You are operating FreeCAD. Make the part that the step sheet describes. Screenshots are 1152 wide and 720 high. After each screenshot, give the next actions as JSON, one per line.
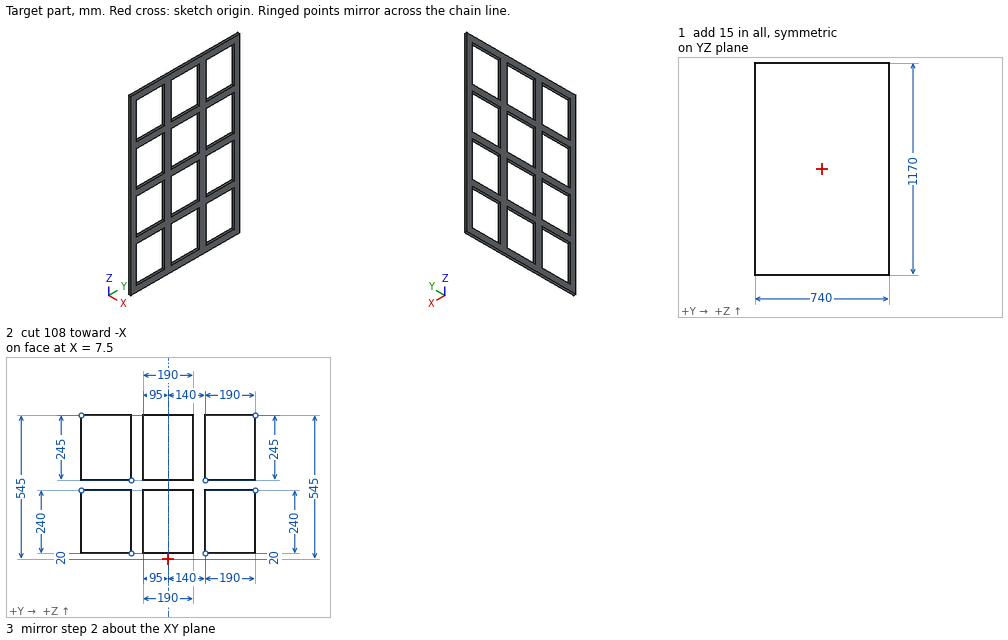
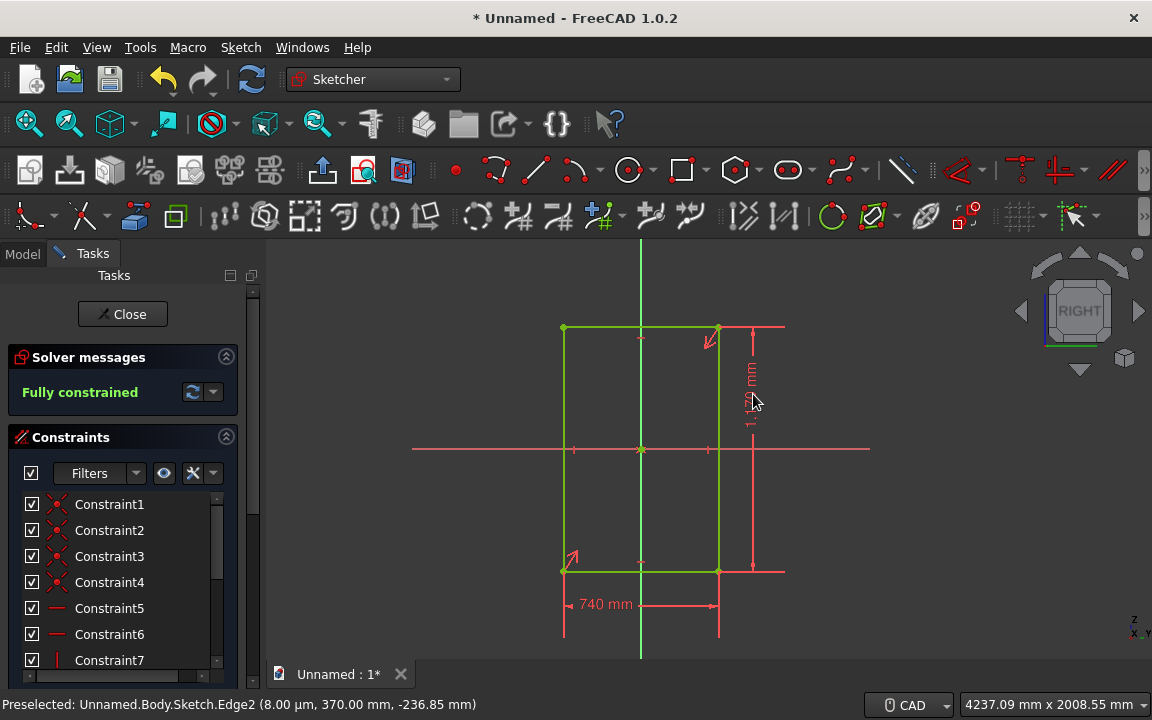
{"action": "left_click", "coordinate": [123, 314]}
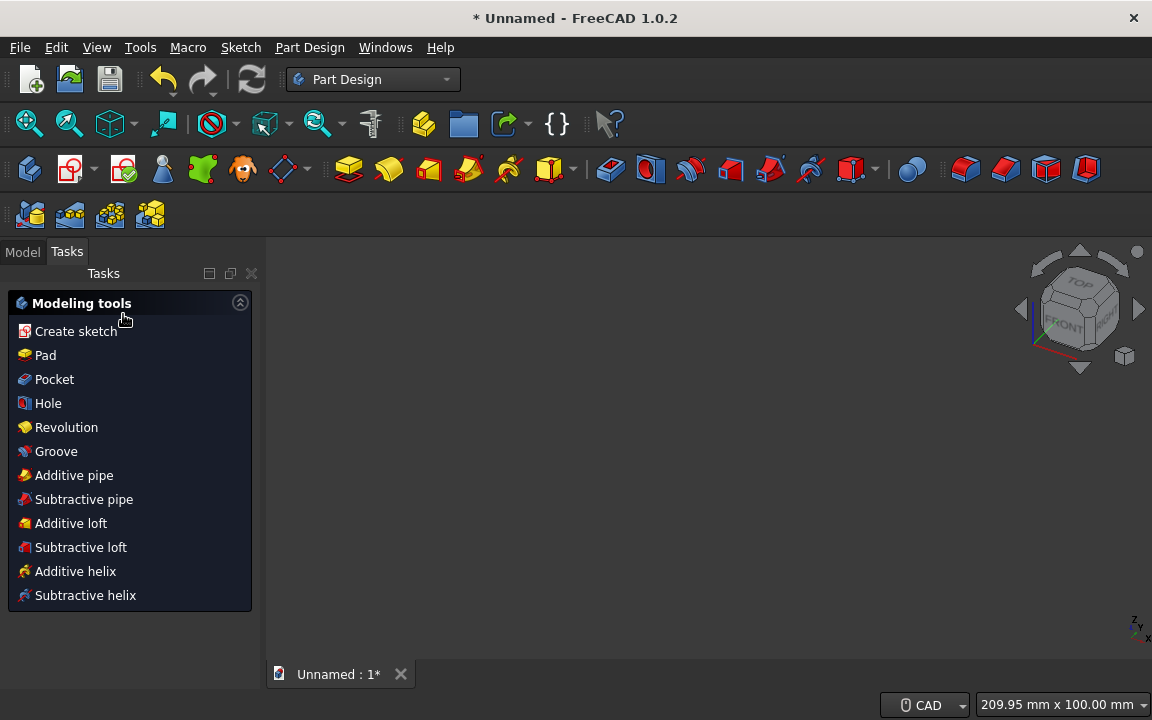
{"action": "left_click", "coordinate": [350, 170]}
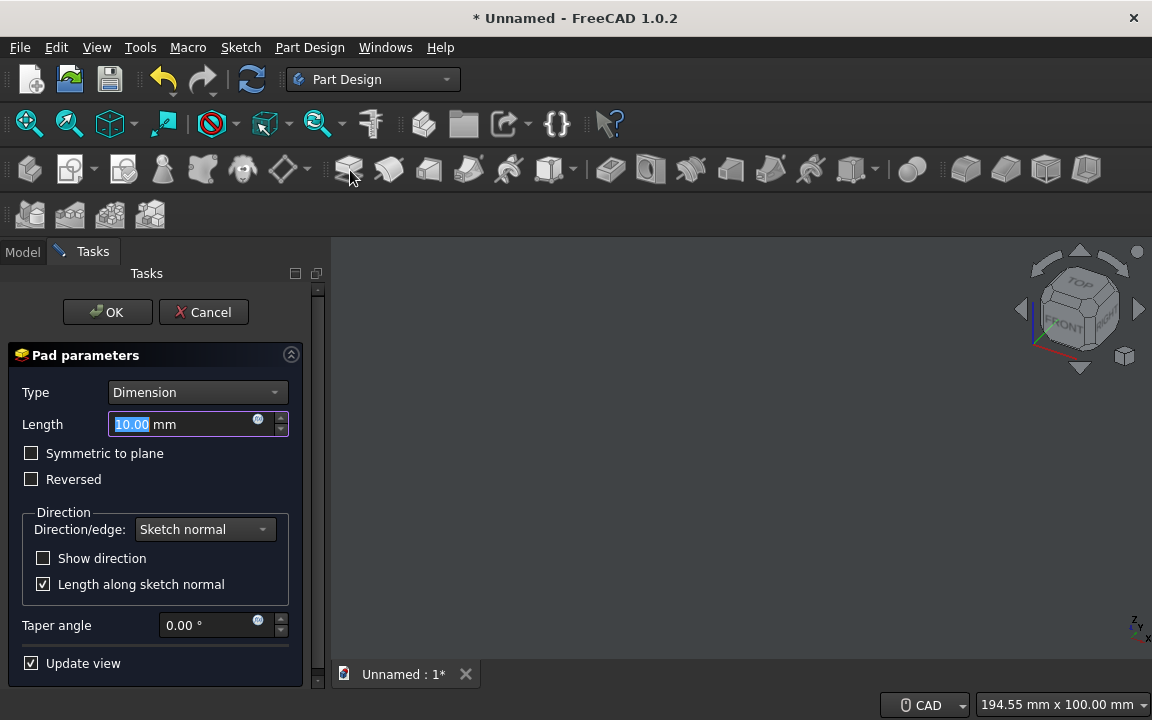
{"action": "type", "text": "15"}
{"action": "key", "text": "Tab"}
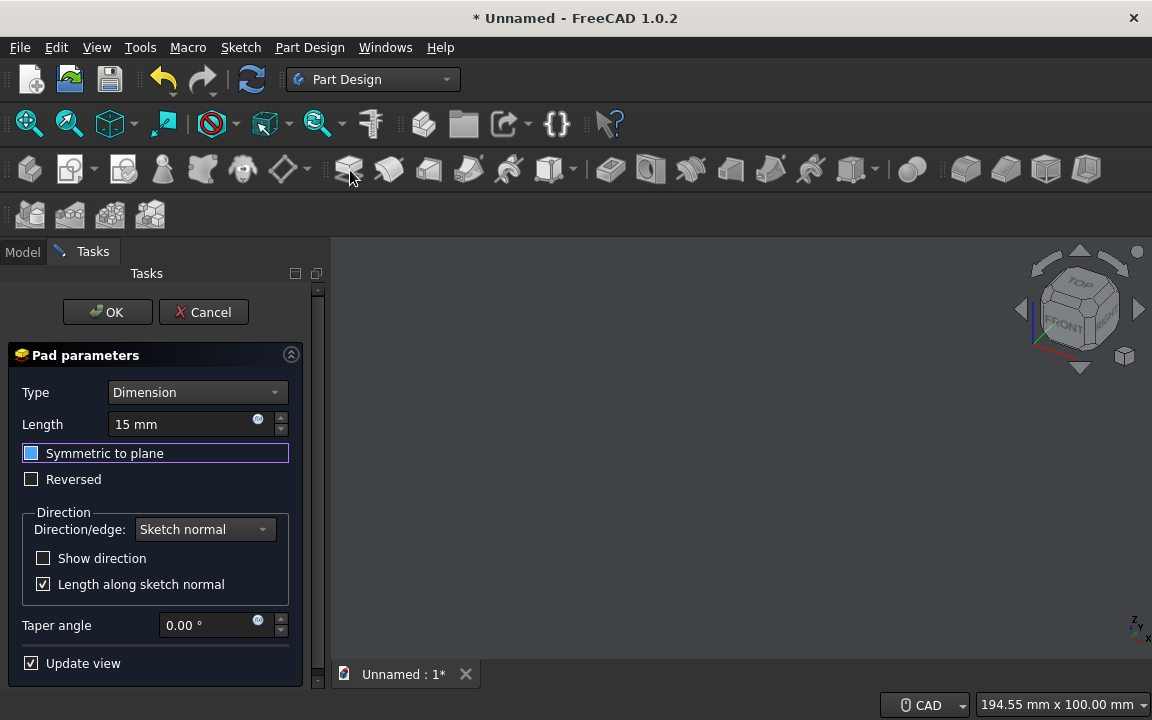
{"action": "left_click", "coordinate": [30, 453]}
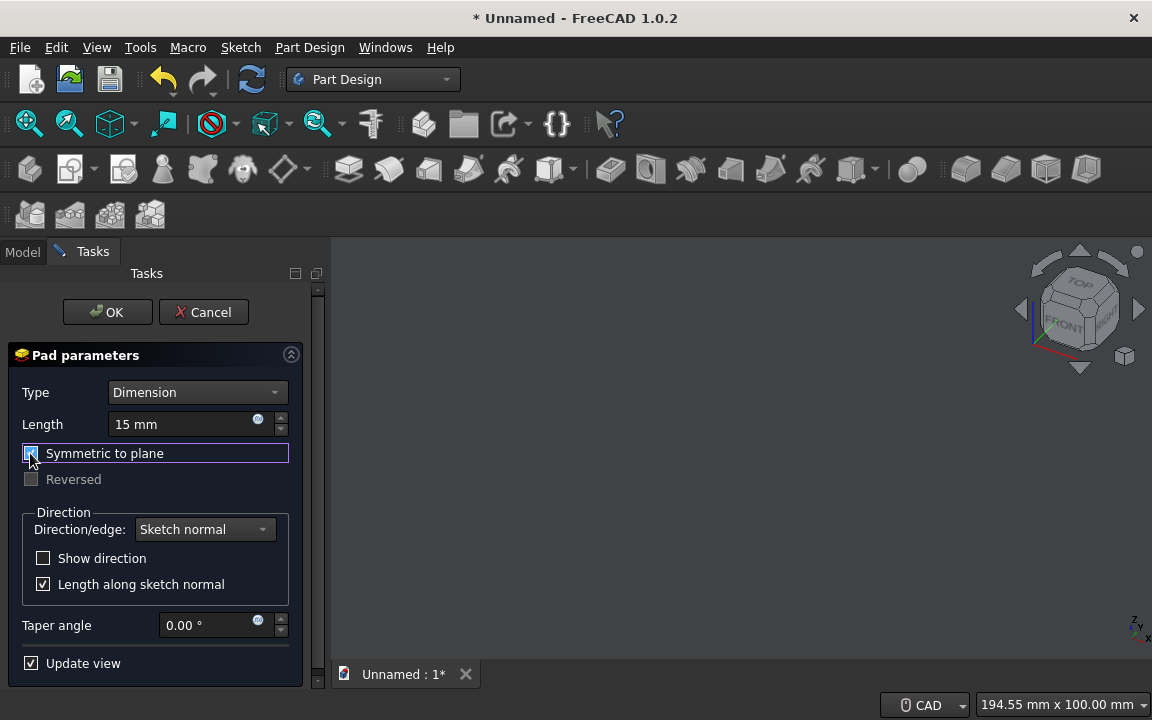
{"action": "left_click", "coordinate": [108, 312]}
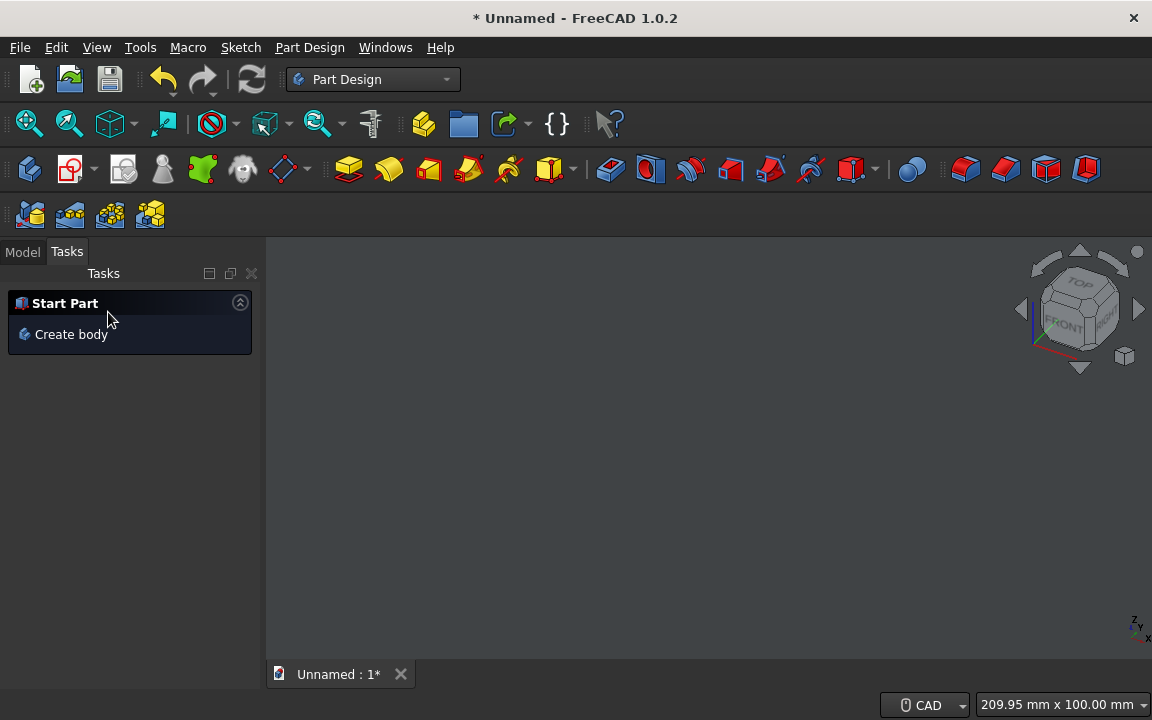
{"action": "left_click", "coordinate": [30, 124]}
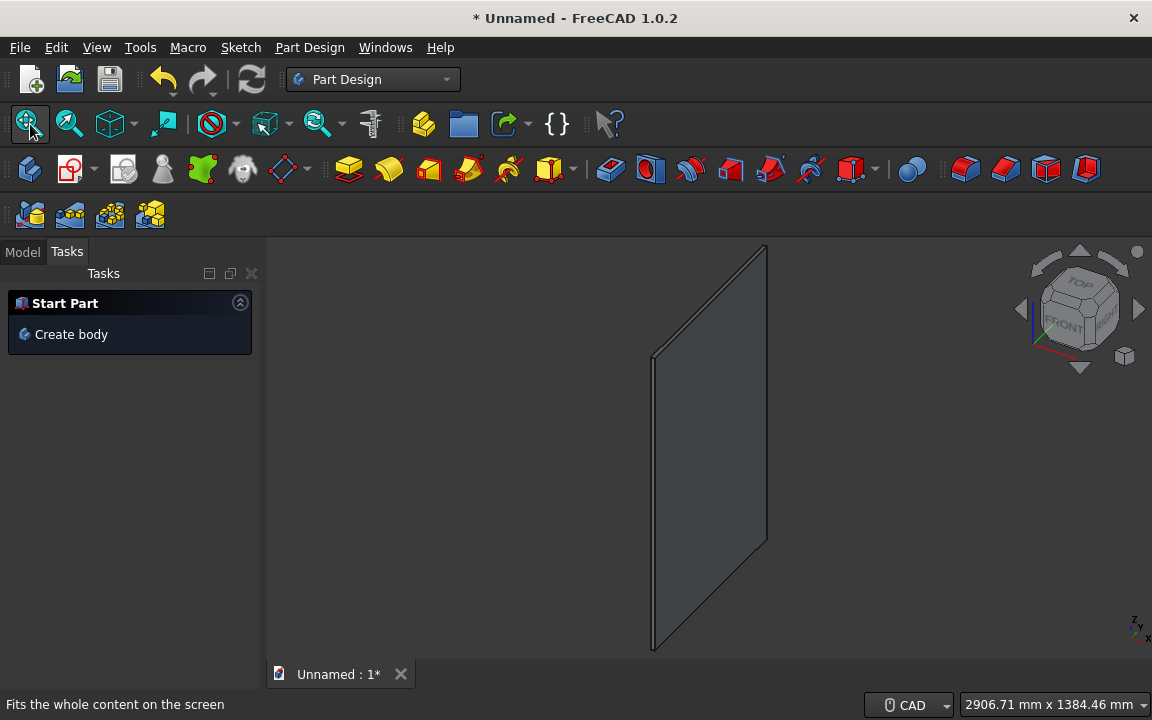
{"action": "left_click", "coordinate": [711, 489]}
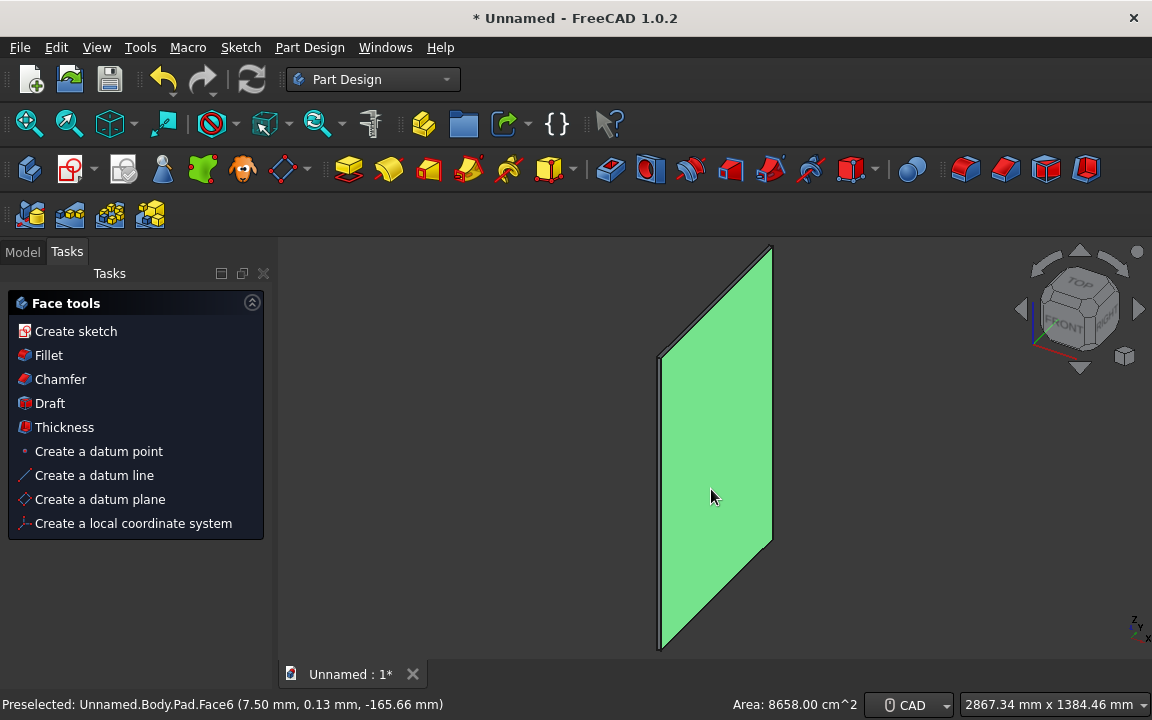
{"action": "left_click", "coordinate": [70, 170]}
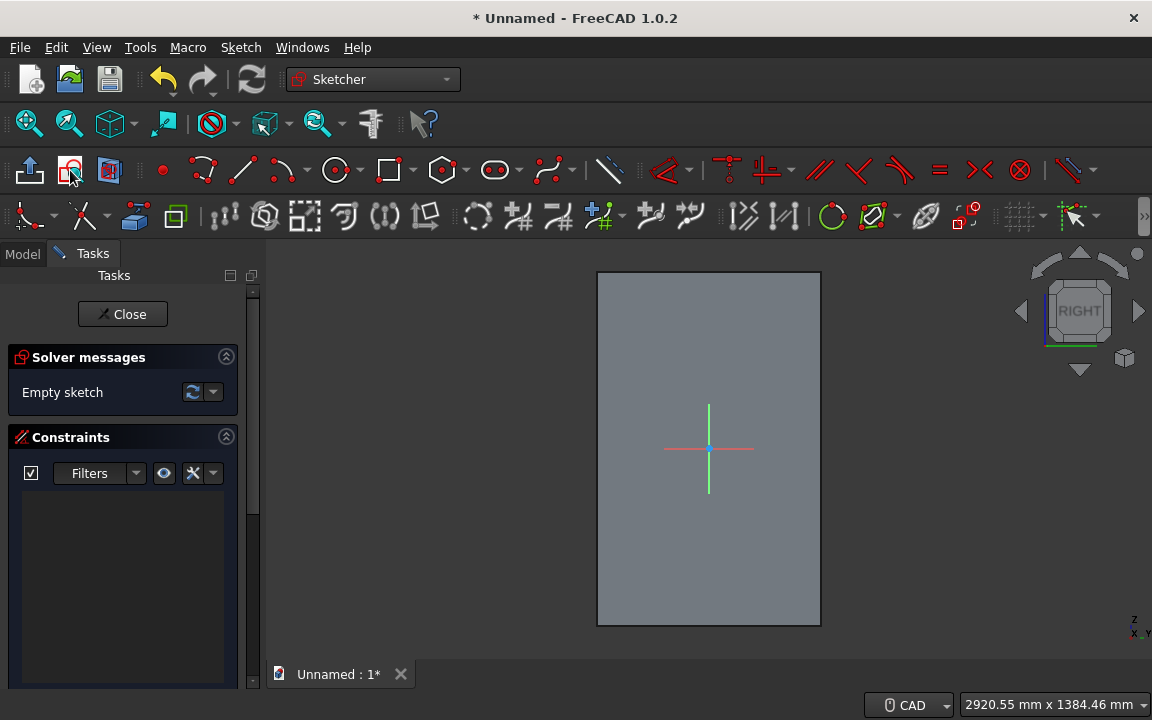
{"action": "scroll", "coordinate": [331, 631], "scroll_direction": "down", "scroll_amount": 1}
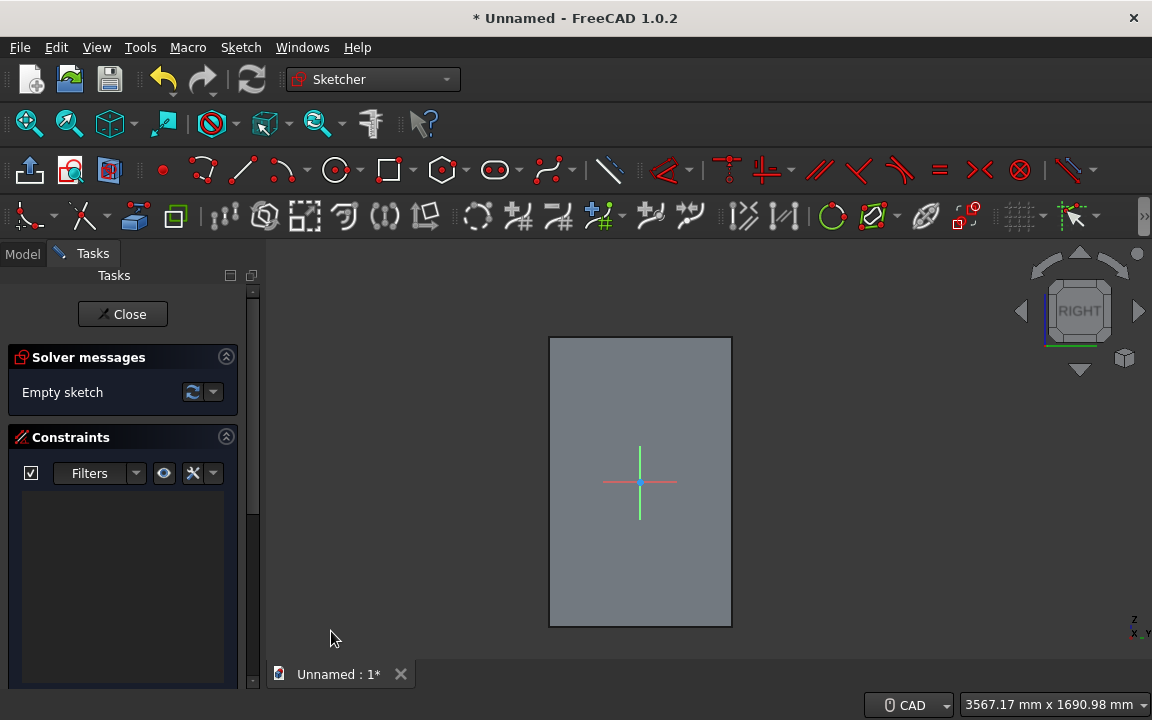
{"action": "scroll", "coordinate": [640, 372], "scroll_direction": "up", "scroll_amount": 3}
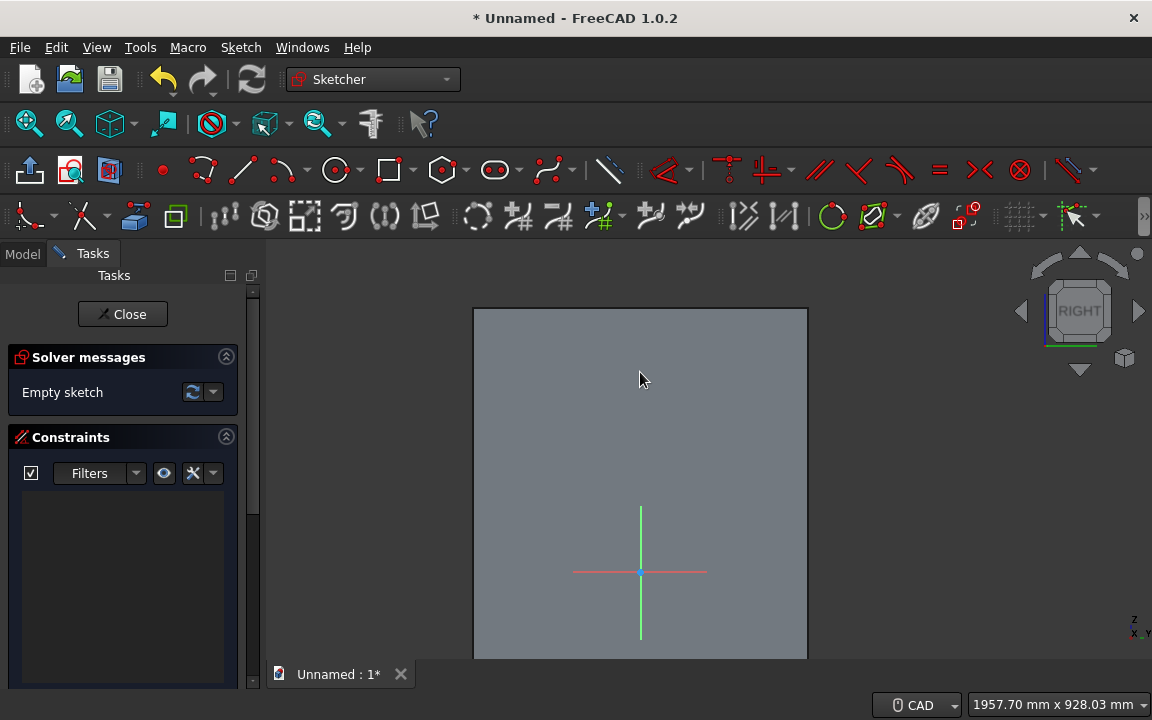
{"action": "key", "text": "g r"}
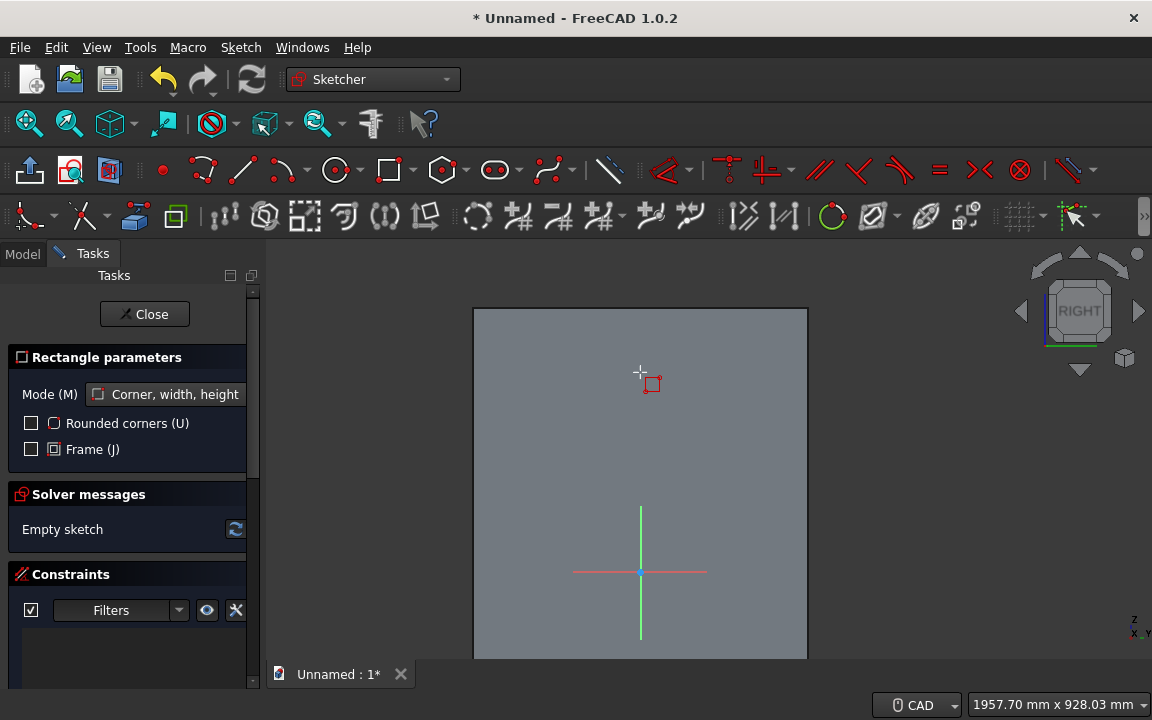
{"action": "left_click", "coordinate": [704, 326]}
{"action": "left_click", "coordinate": [790, 437]}